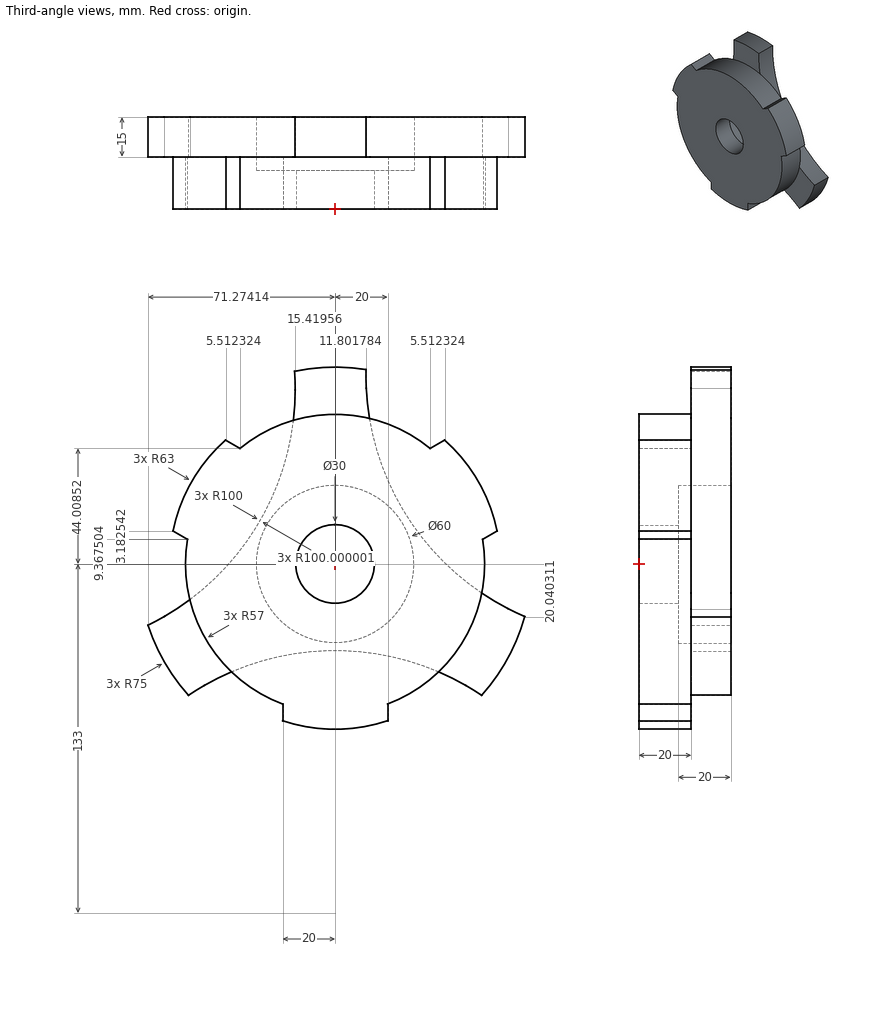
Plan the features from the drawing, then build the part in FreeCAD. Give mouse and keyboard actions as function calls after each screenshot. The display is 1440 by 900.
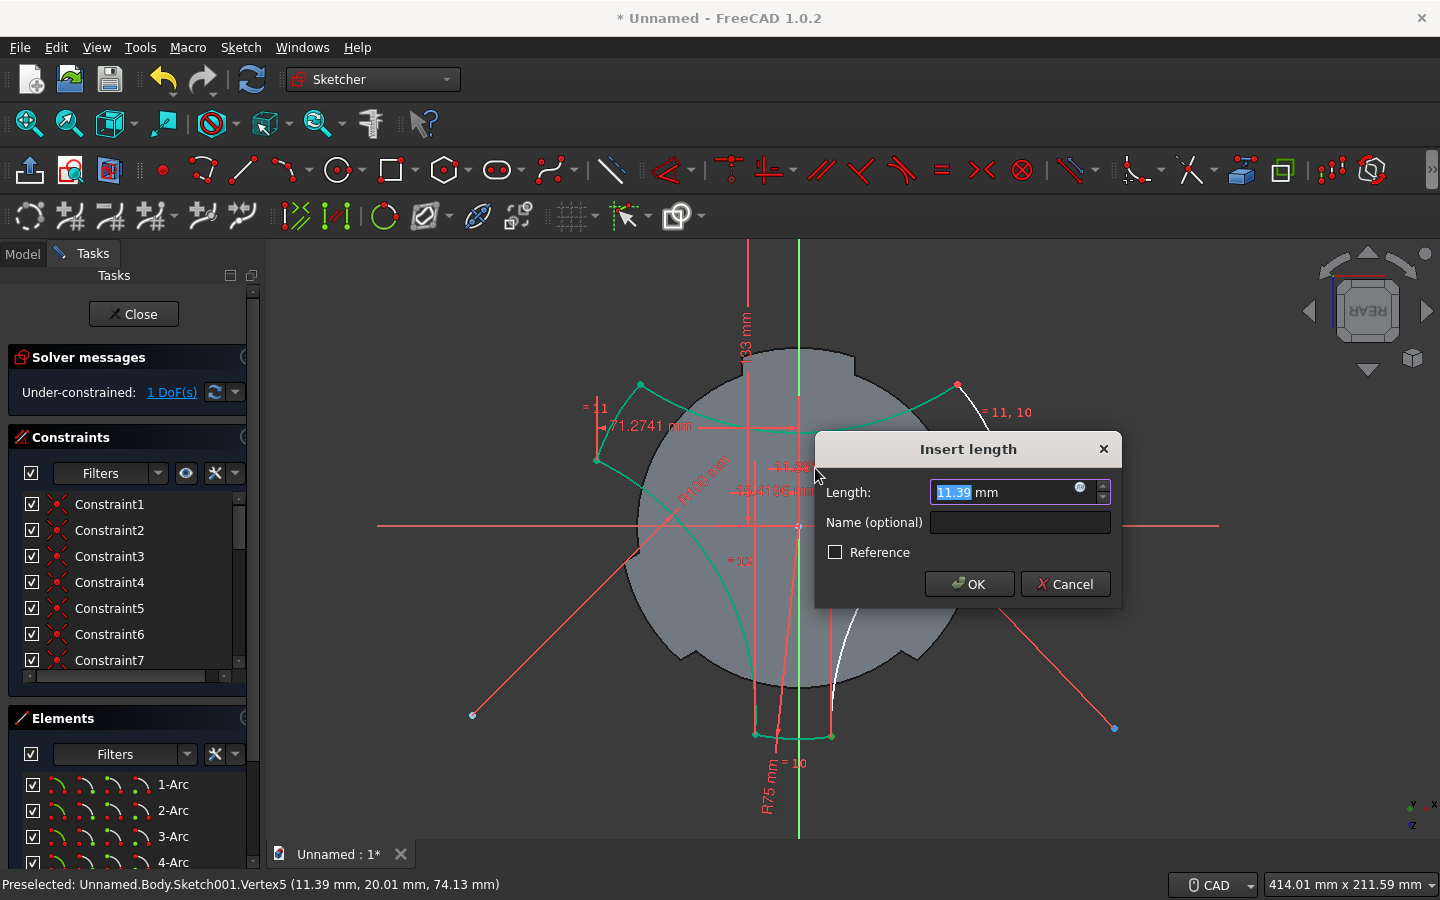
text(11.801784)
key(Return)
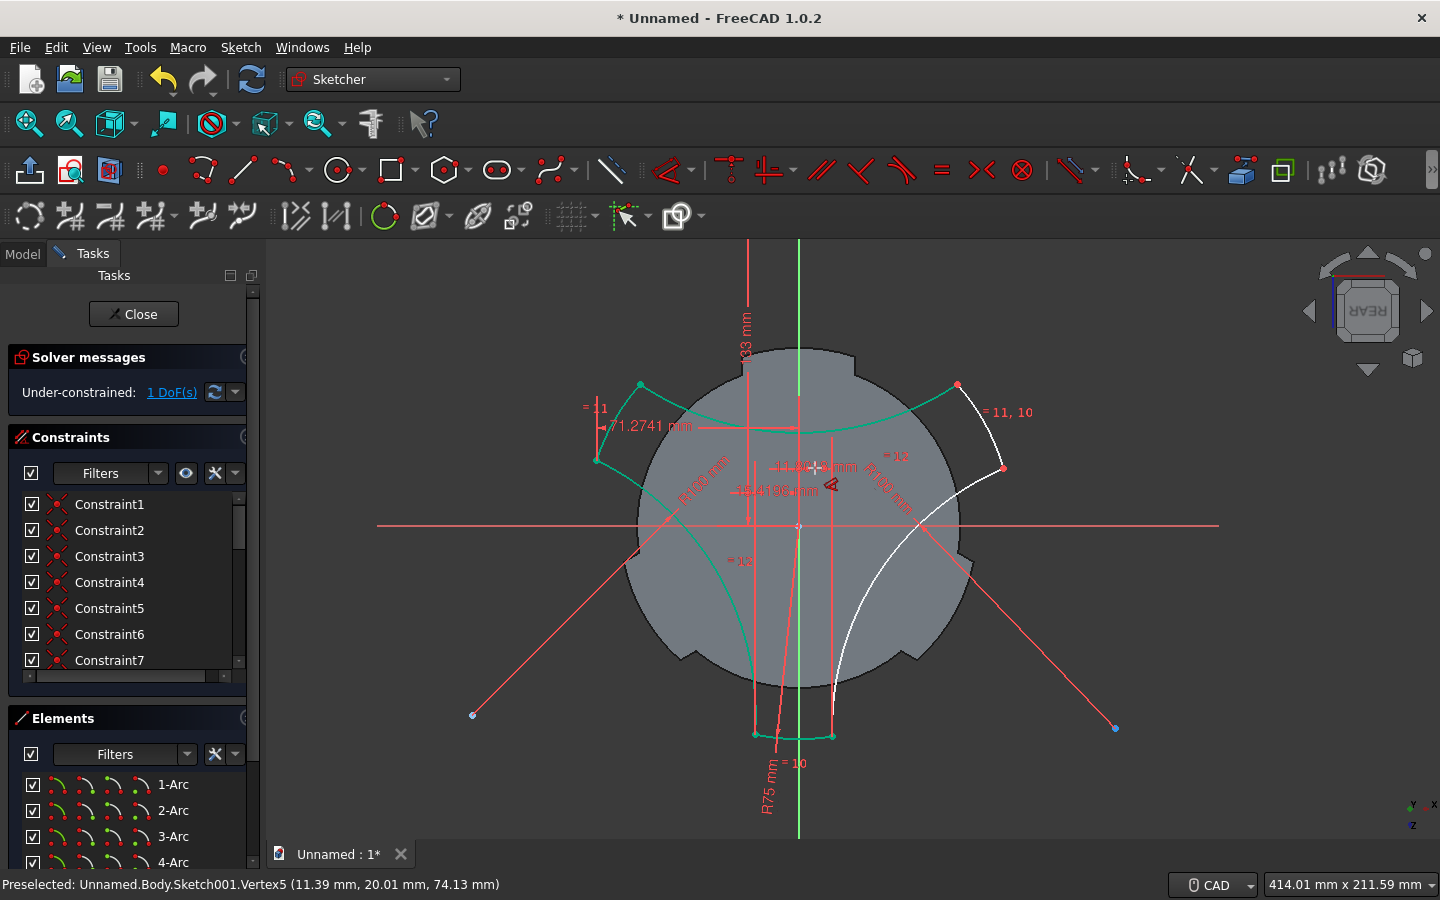
click(1003, 469)
click(1037, 497)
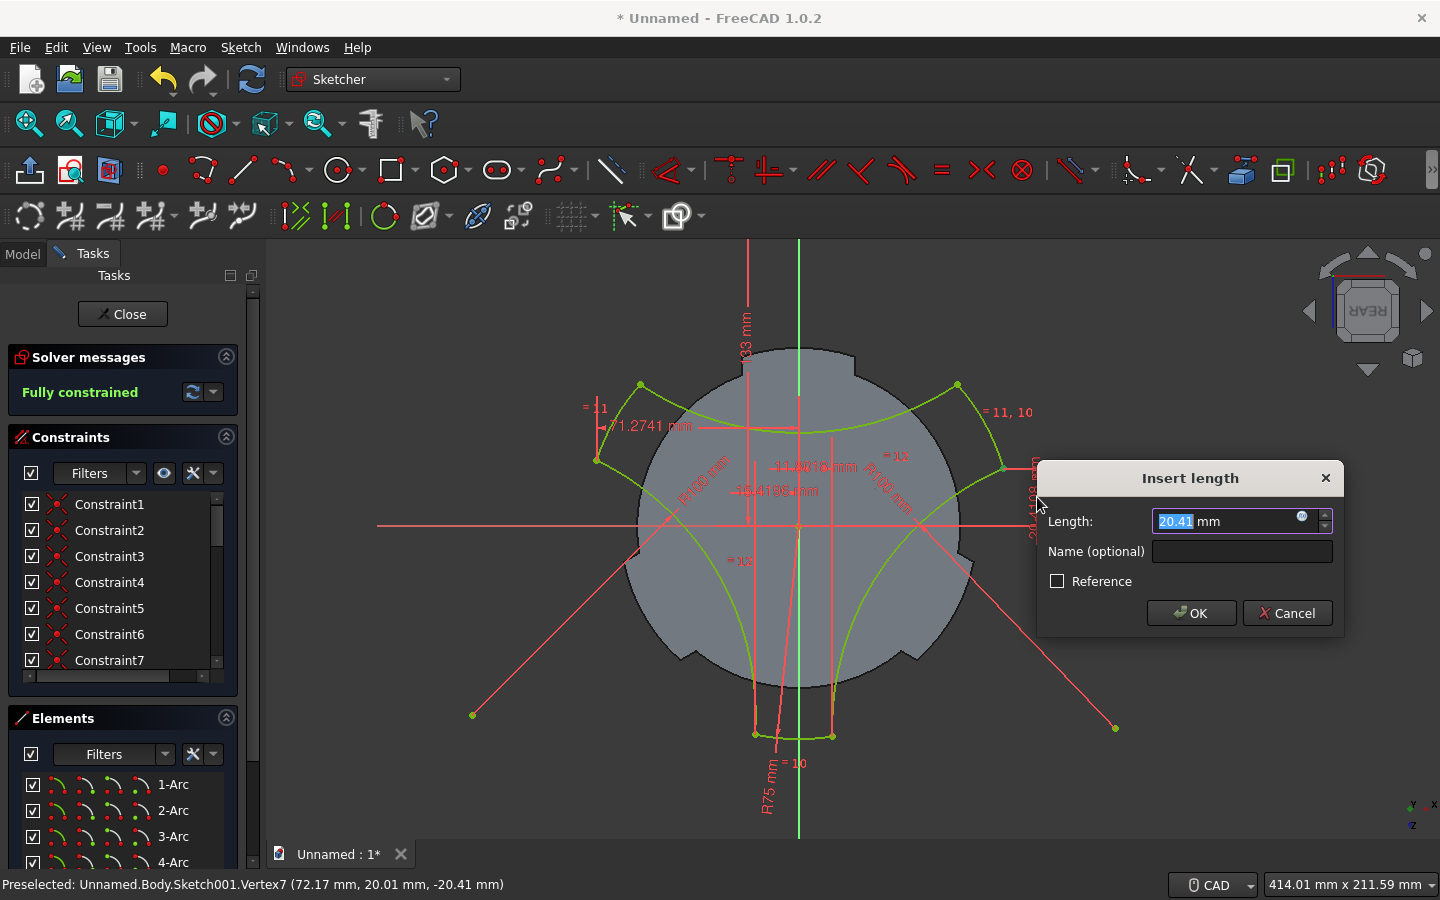
text(20.040311)
key(Return)
key(Escape)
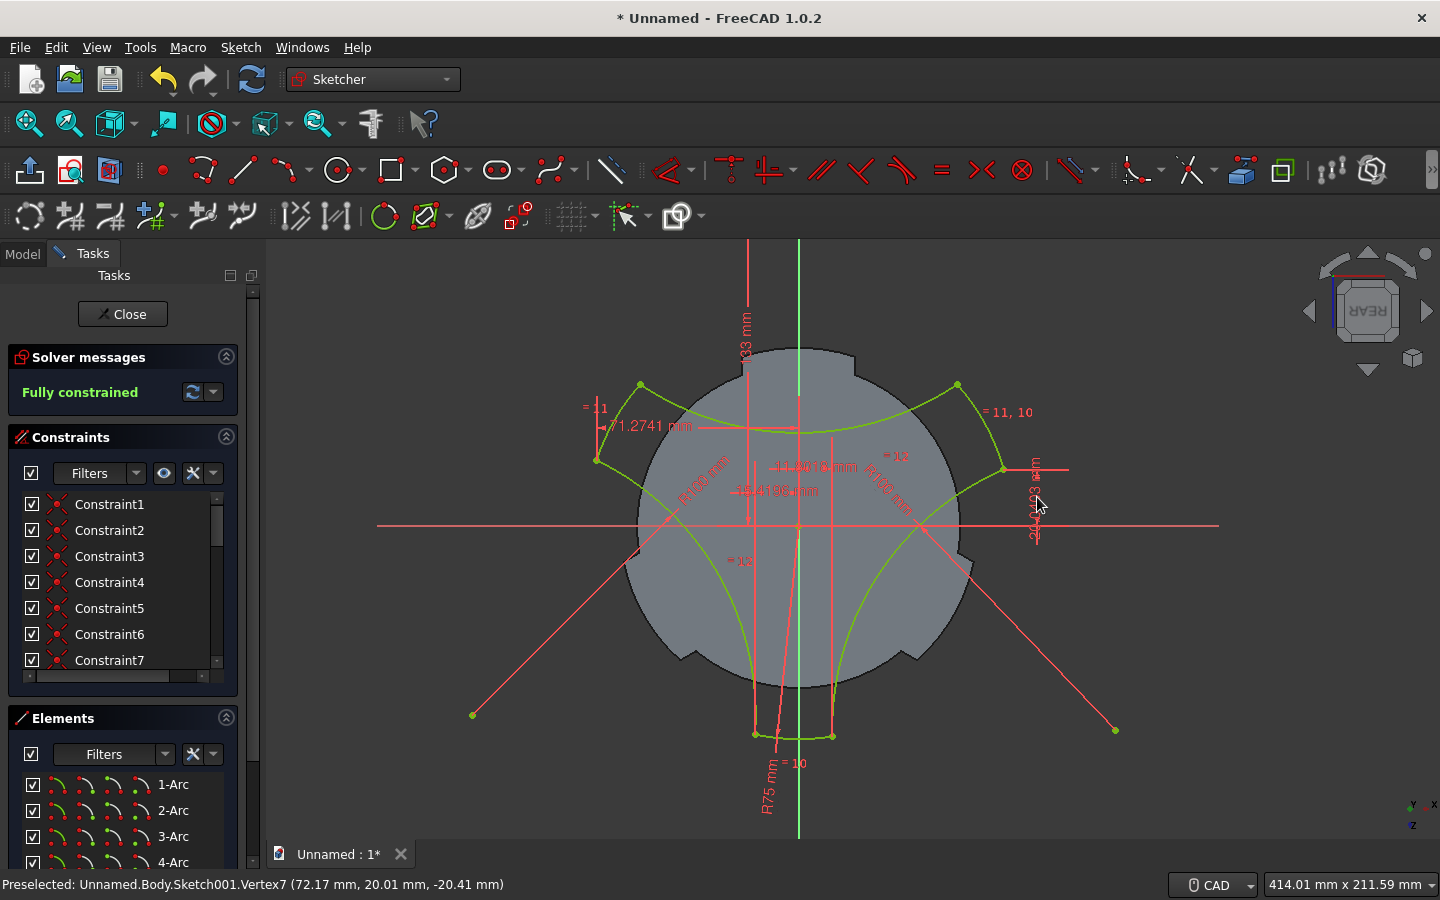
click(123, 314)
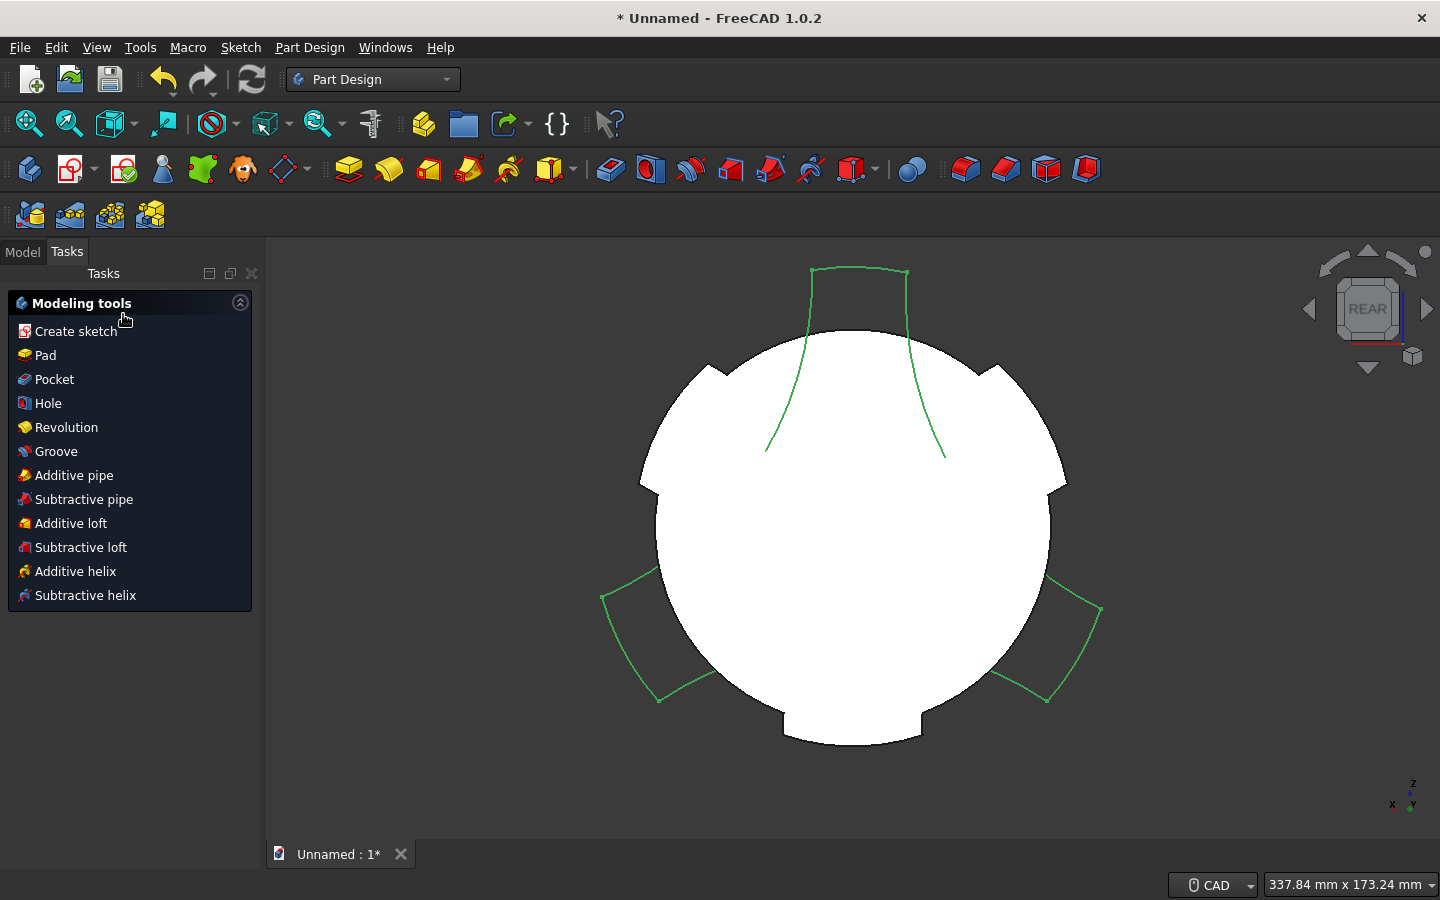
click(350, 170)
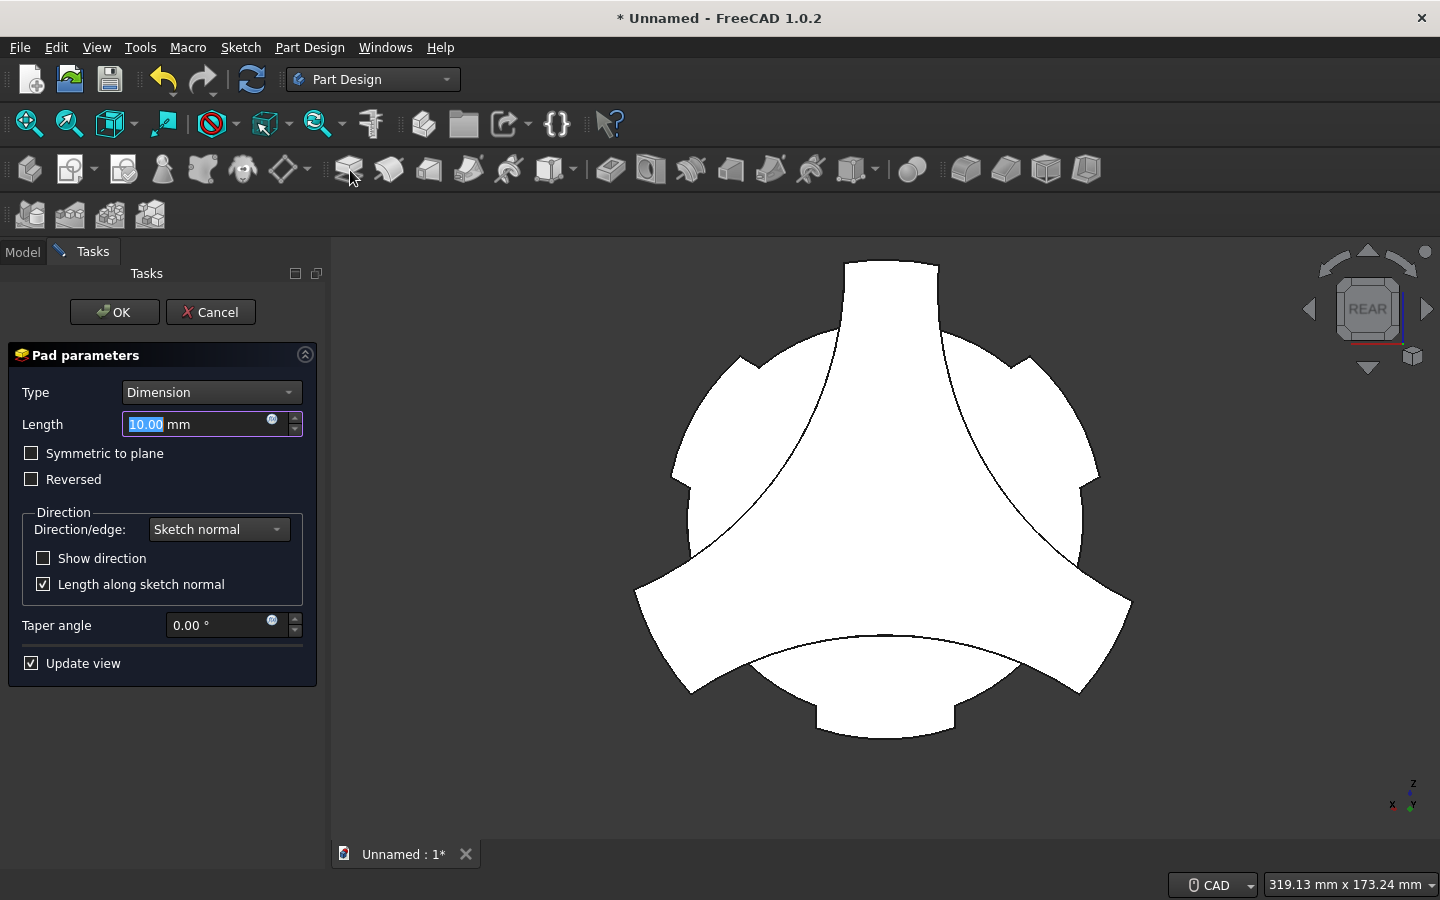
text(15)
key(Tab)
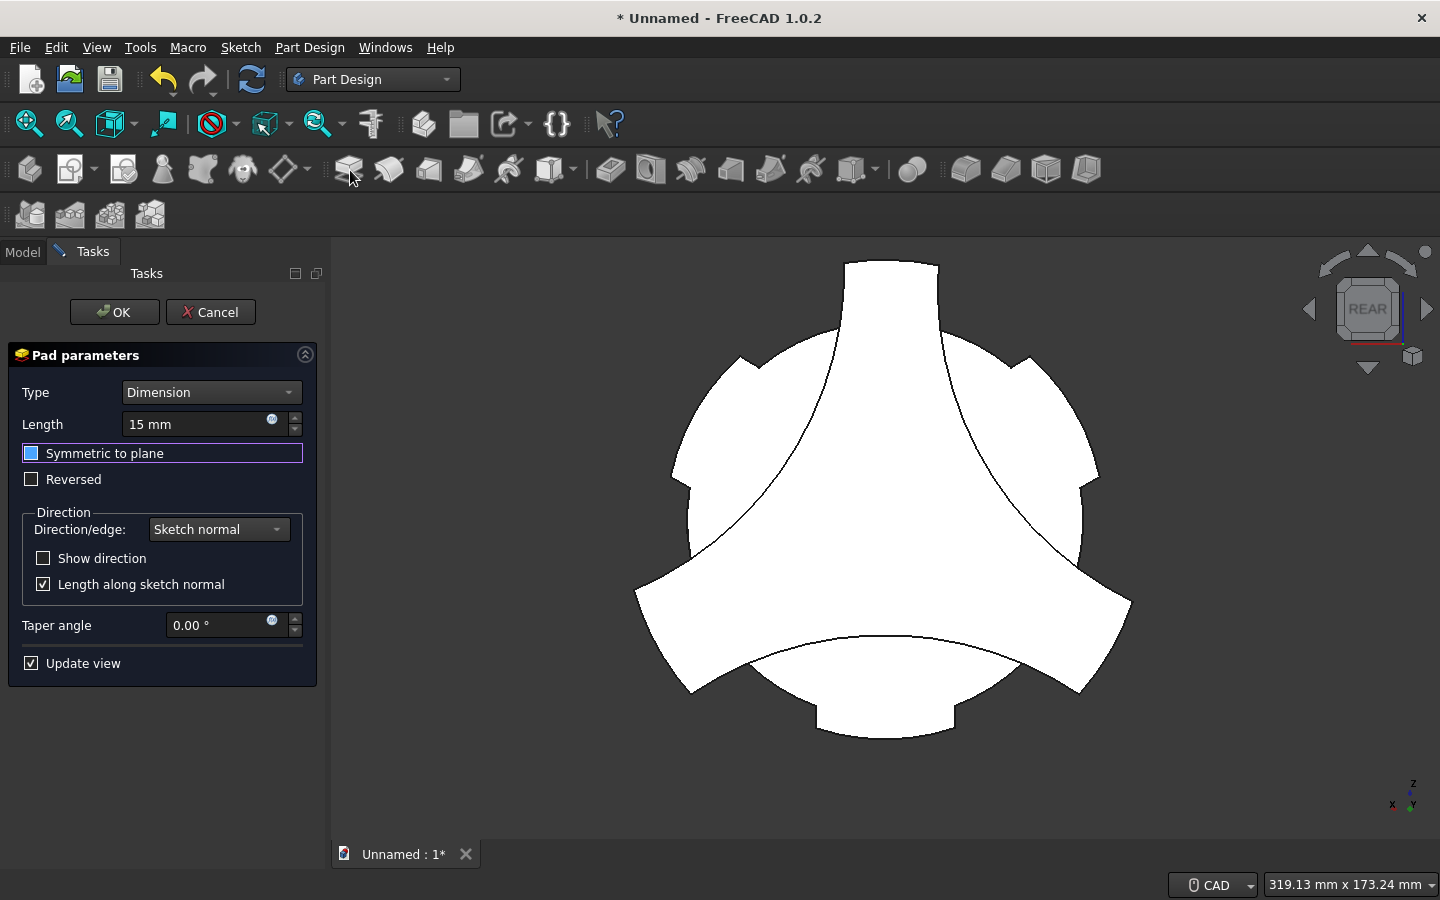
click(115, 312)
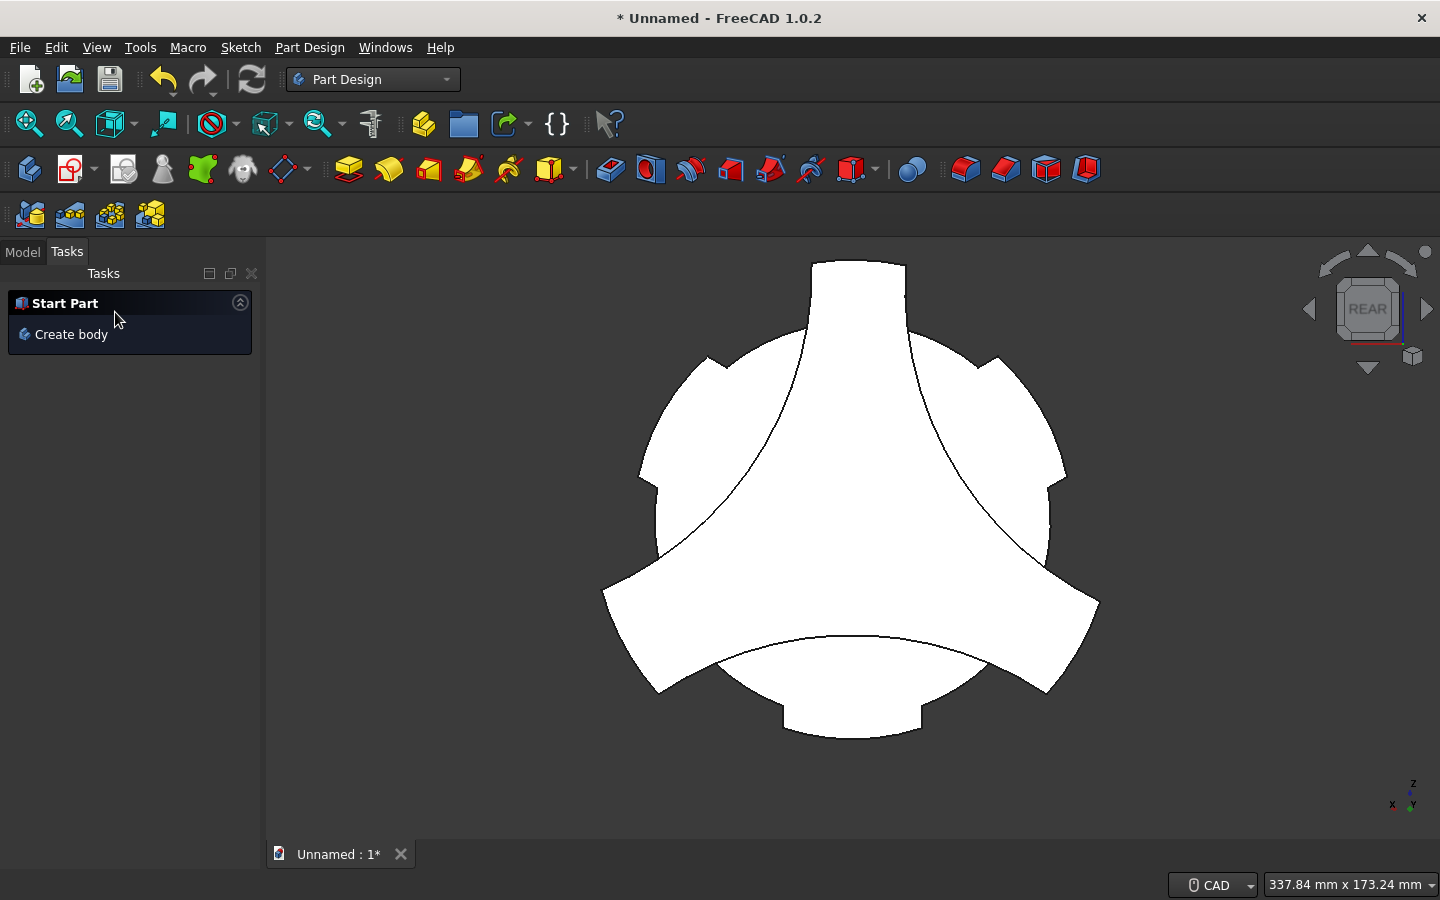
click(851, 538)